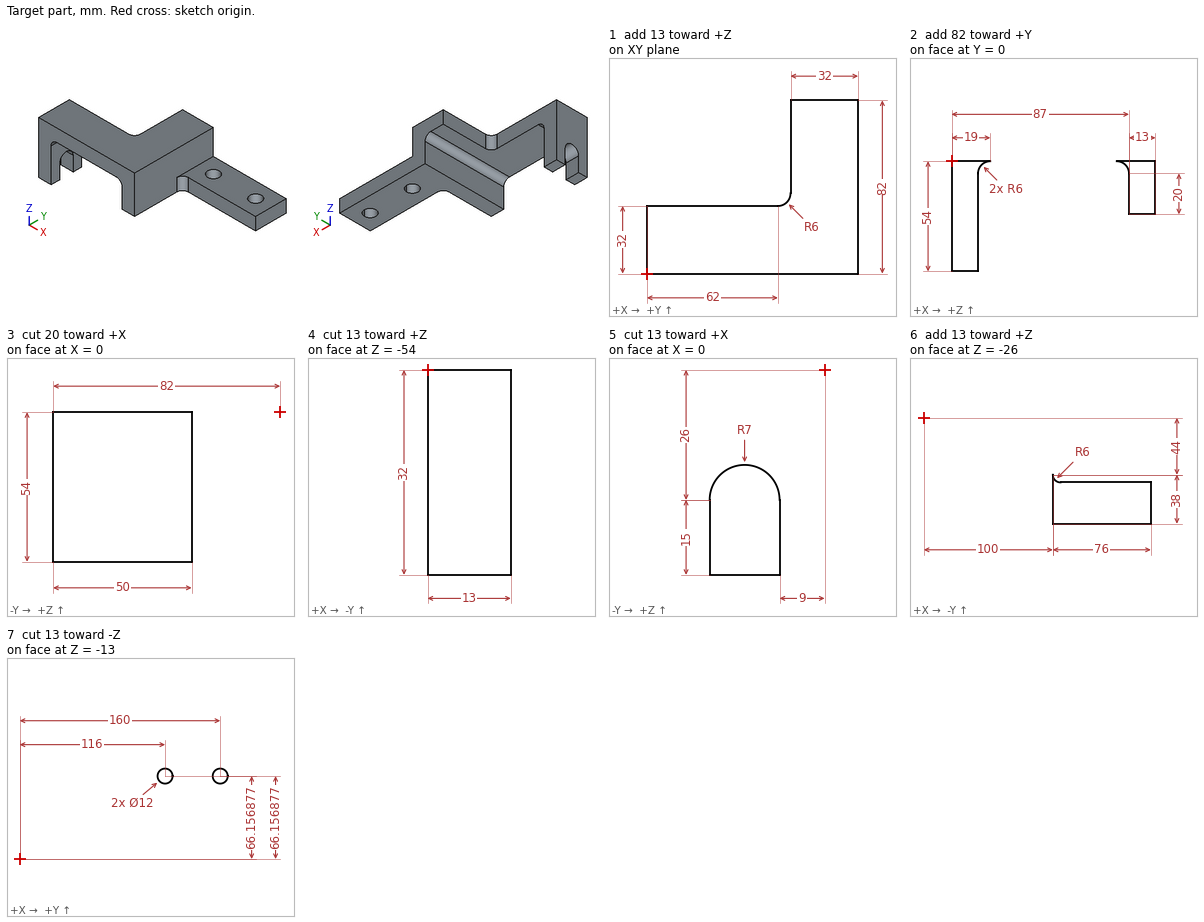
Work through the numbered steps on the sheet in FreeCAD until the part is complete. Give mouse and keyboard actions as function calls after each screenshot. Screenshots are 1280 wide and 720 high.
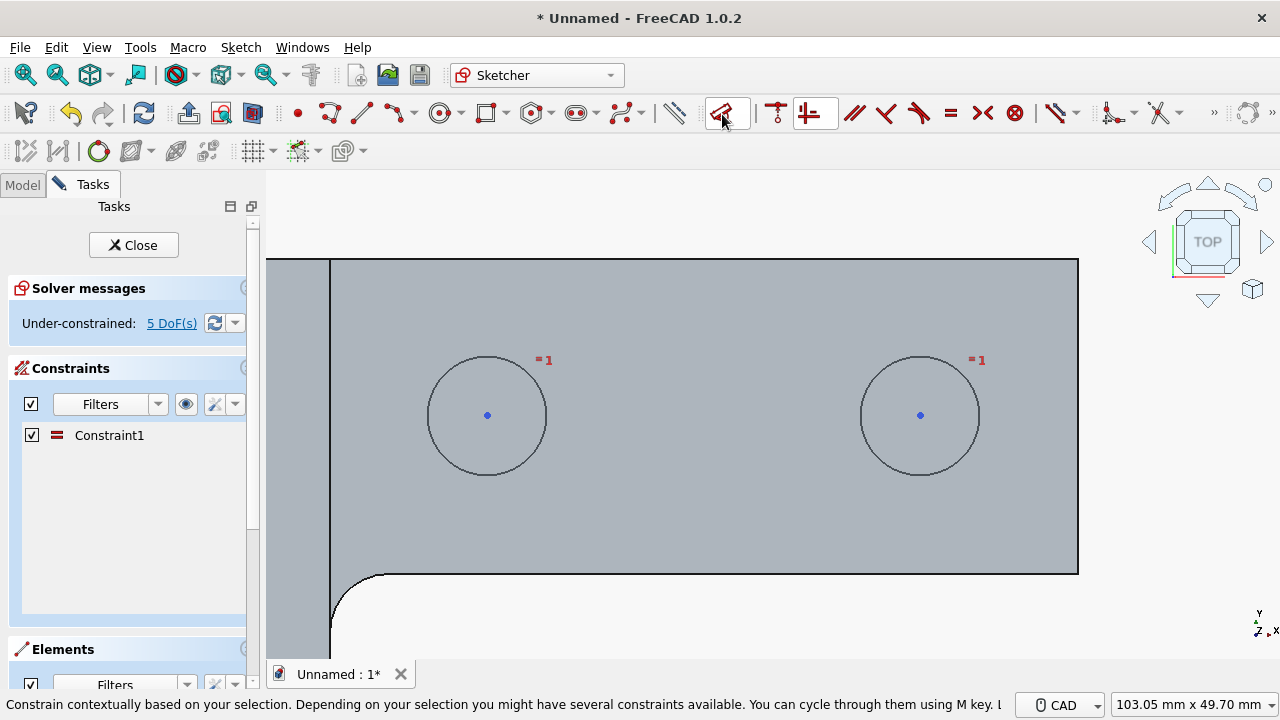
click(529, 374)
click(552, 351)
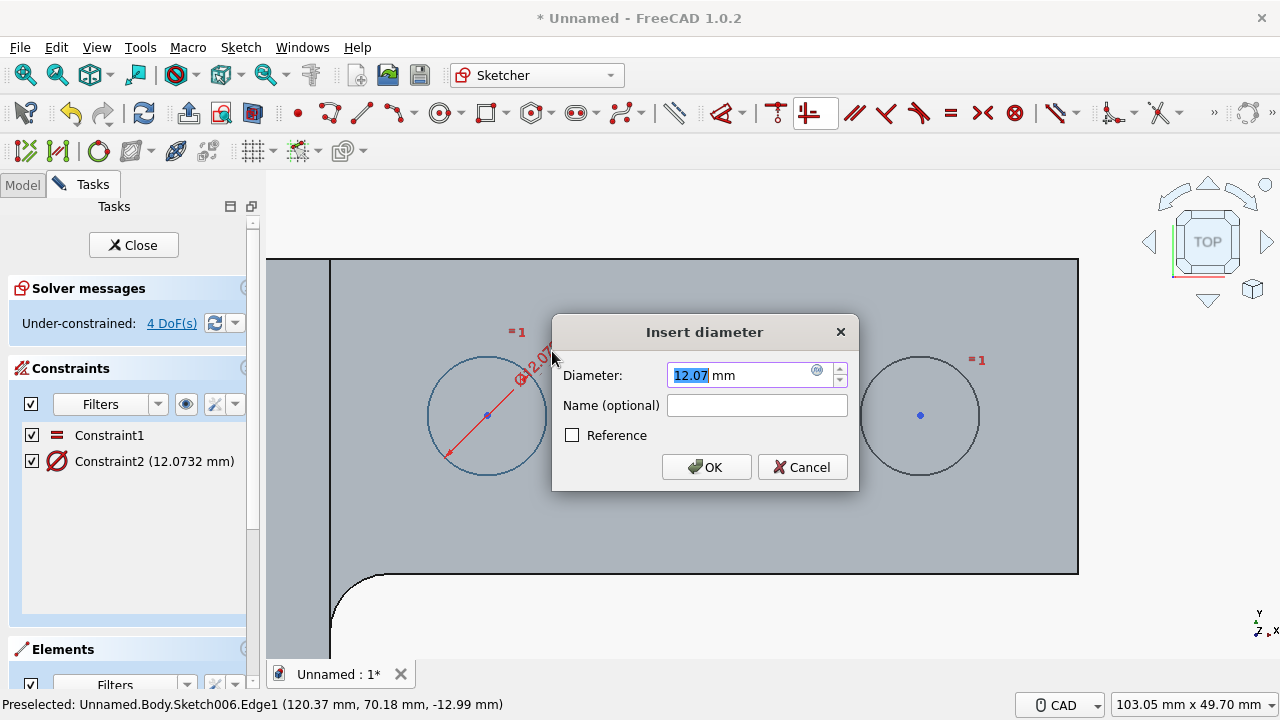
text(12)
key(Return)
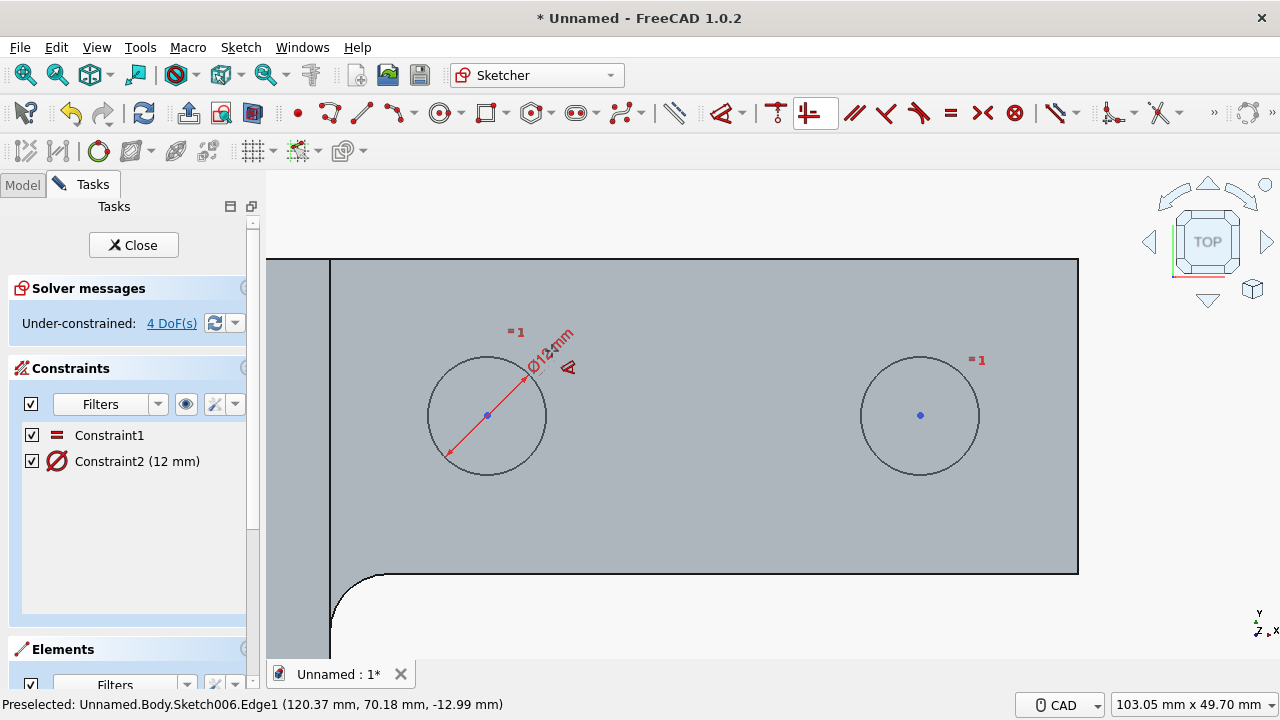
click(487, 416)
click(391, 382)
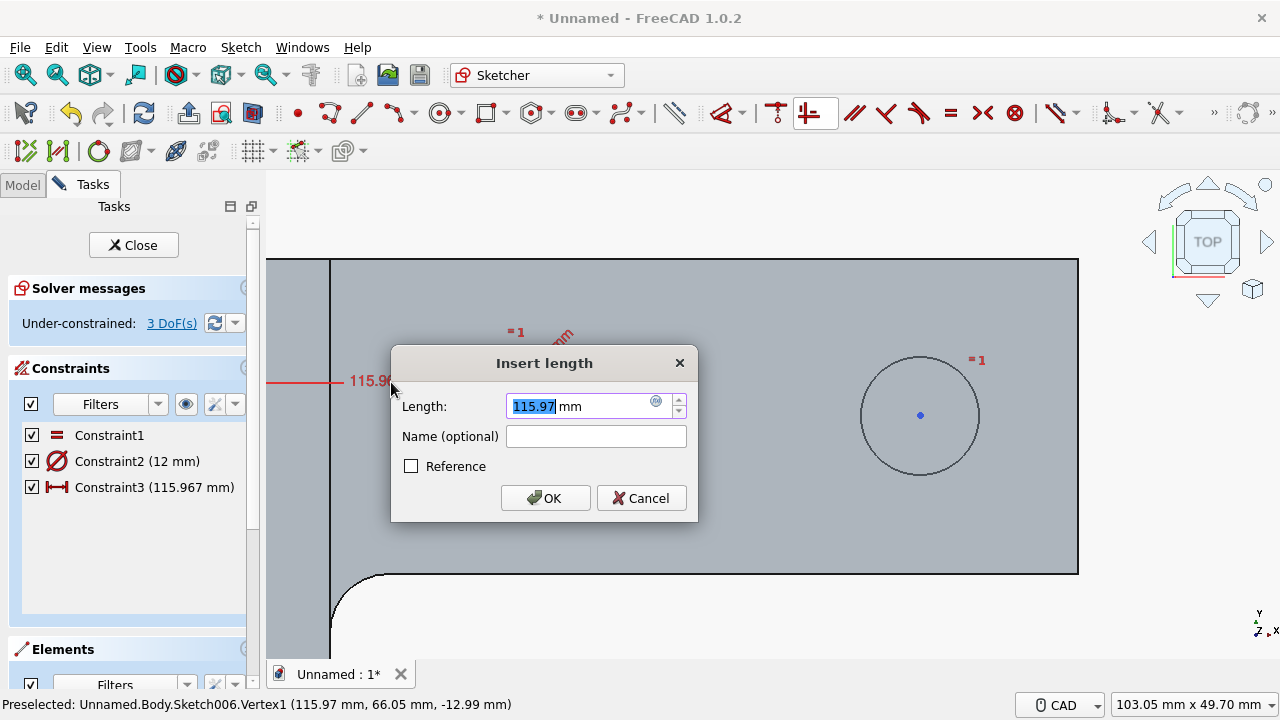
text(116)
key(Return)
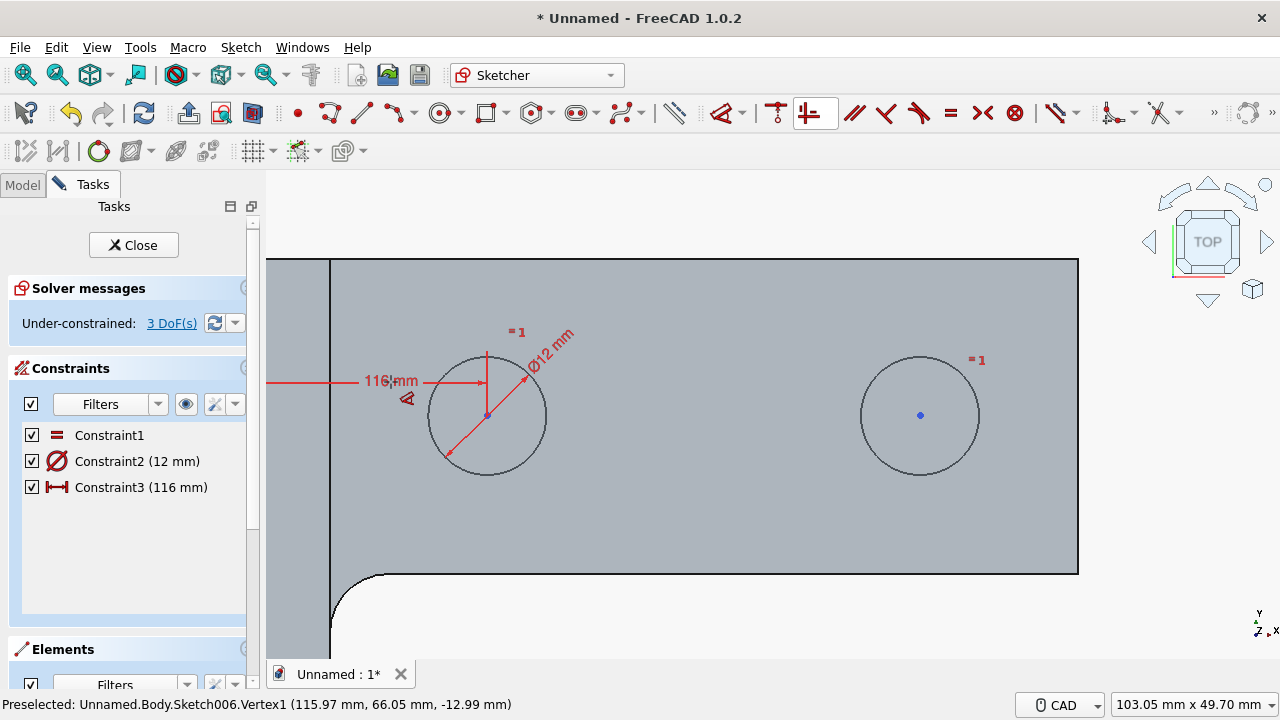
click(920, 416)
click(607, 382)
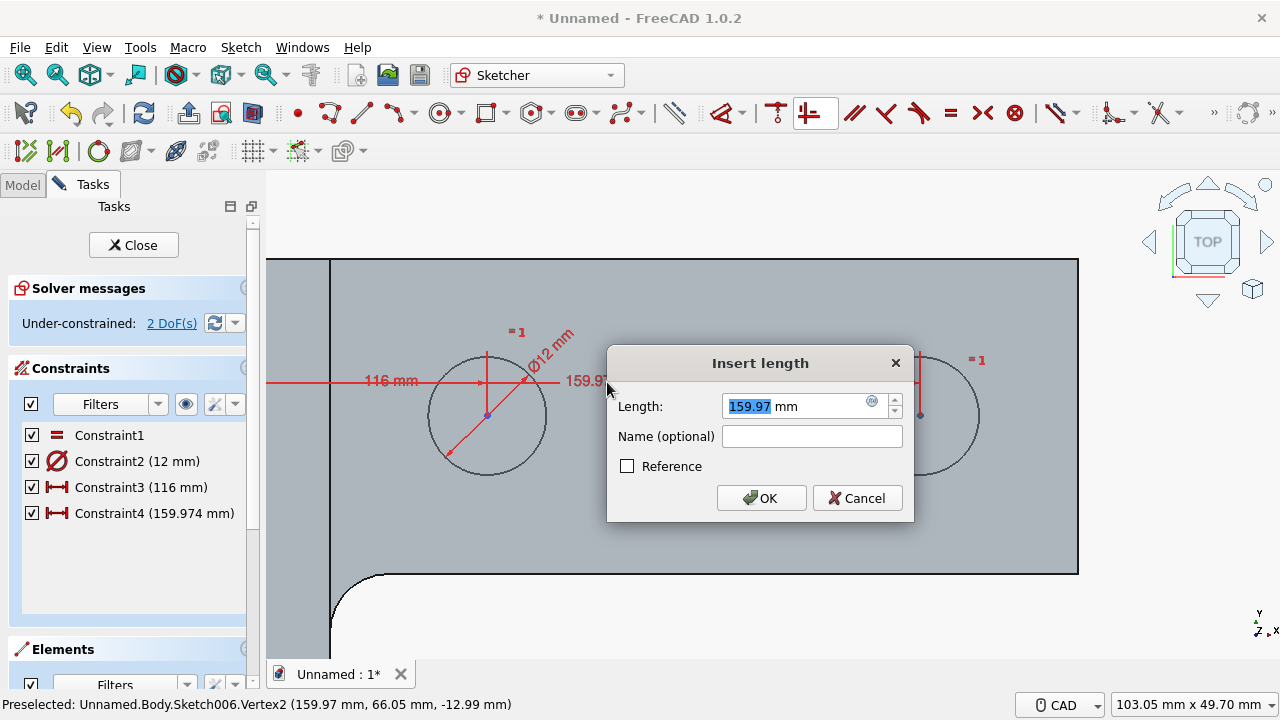
text(160)
key(Return)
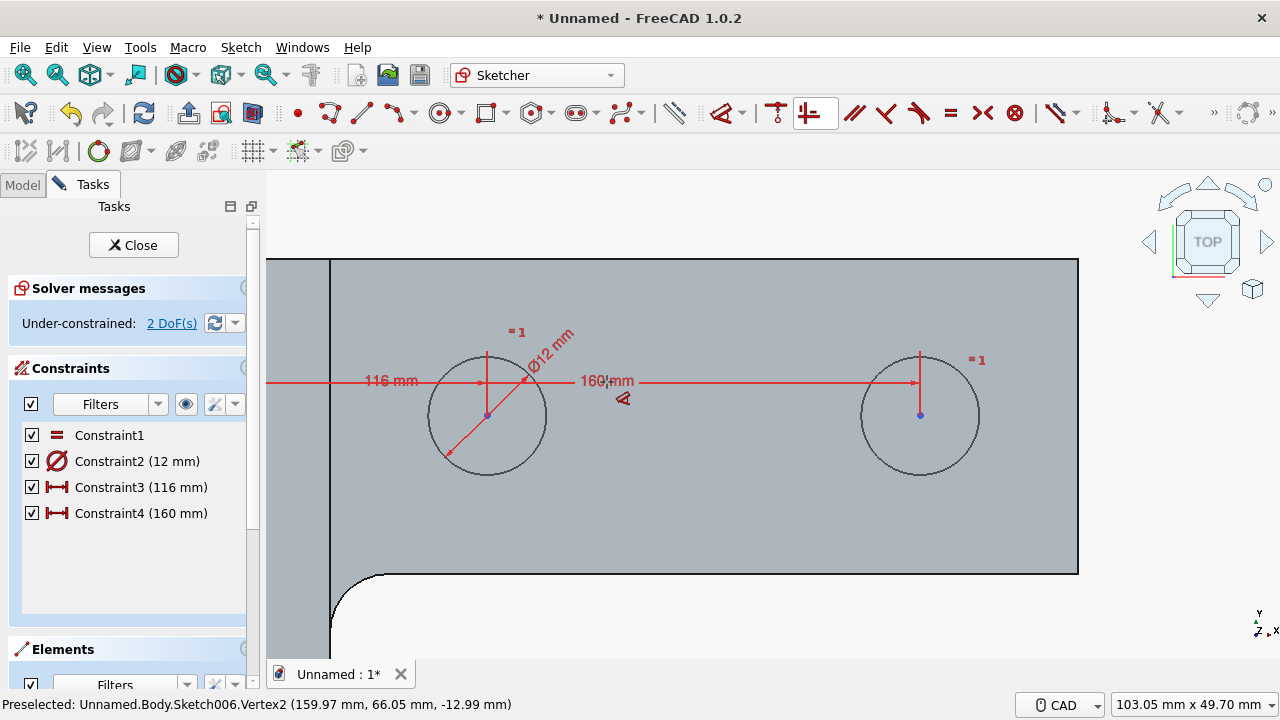
click(487, 416)
click(521, 524)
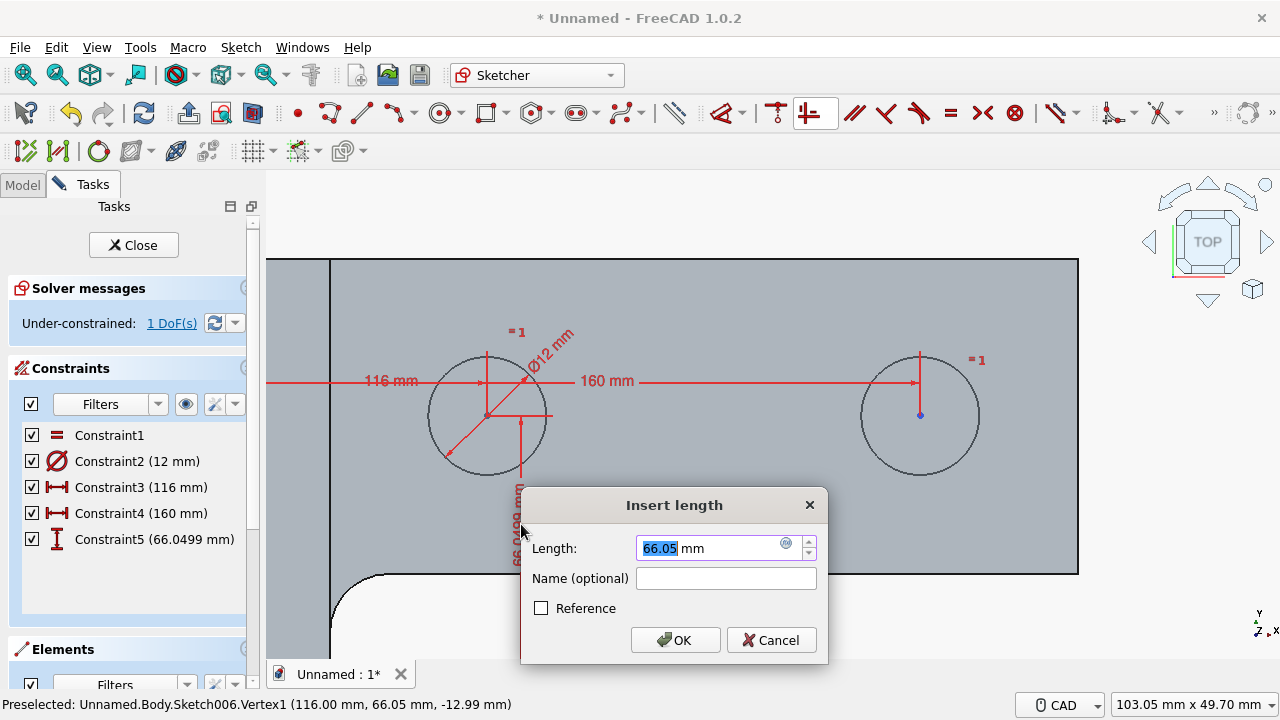
text(66.156877)
key(Return)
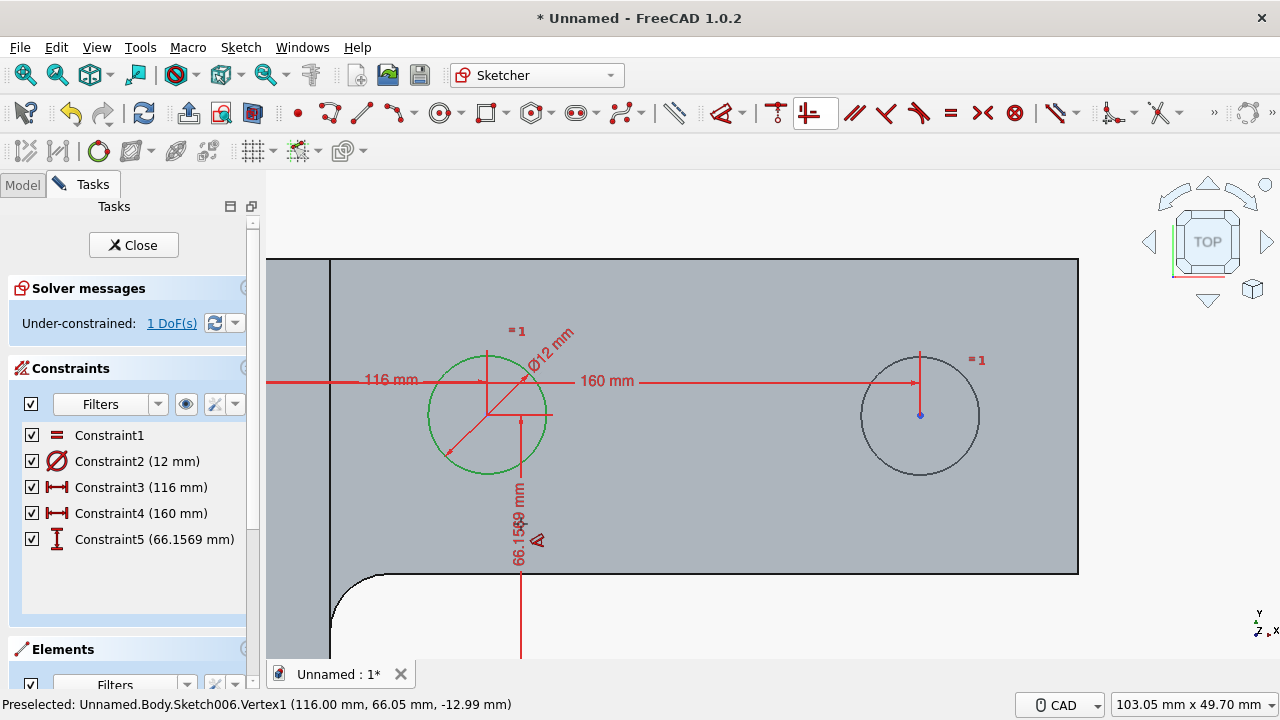
click(920, 416)
click(954, 524)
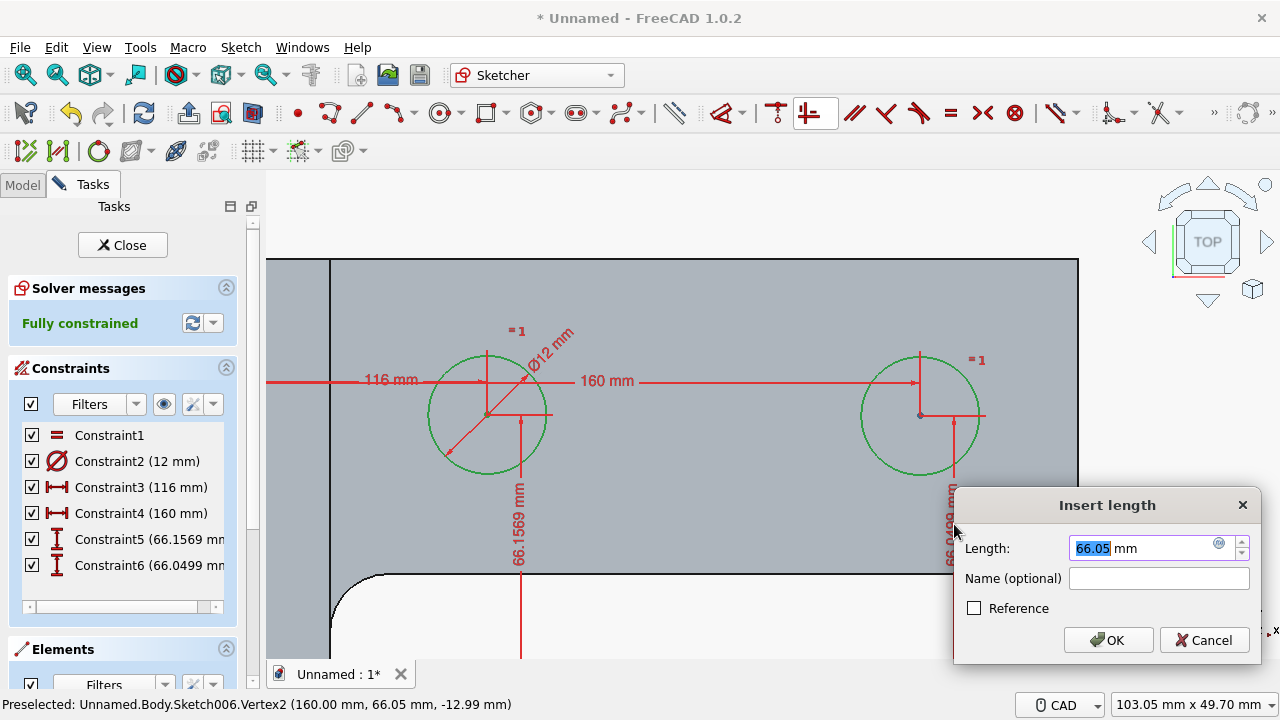
text(66.156877)
key(Return)
key(Escape)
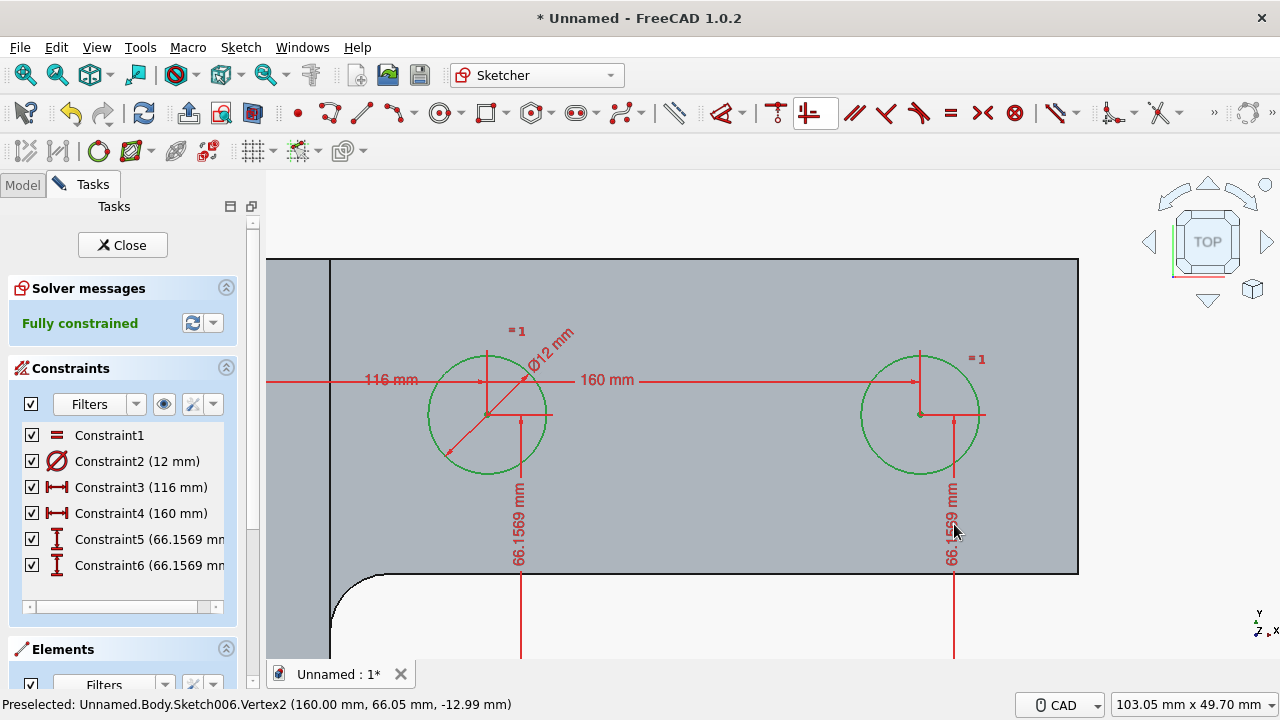
click(123, 245)